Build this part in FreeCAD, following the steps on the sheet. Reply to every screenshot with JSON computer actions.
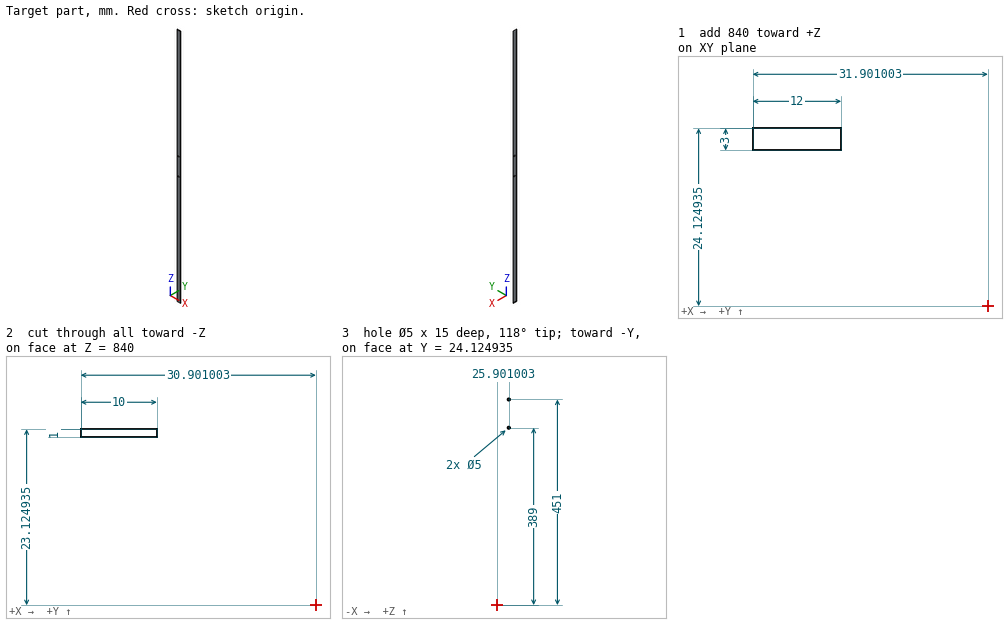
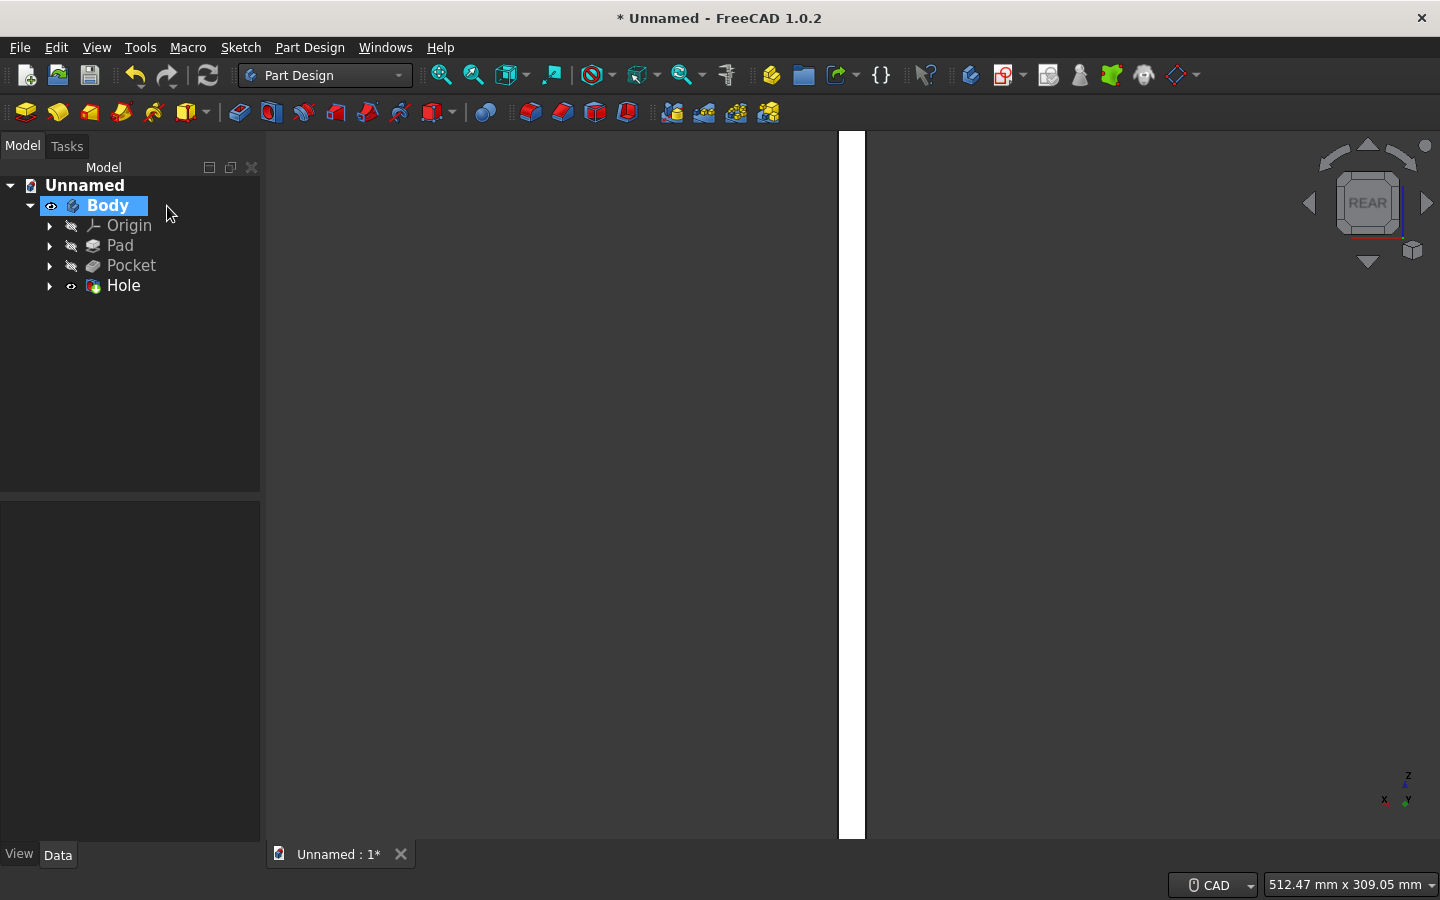
{"action": "key", "text": "0"}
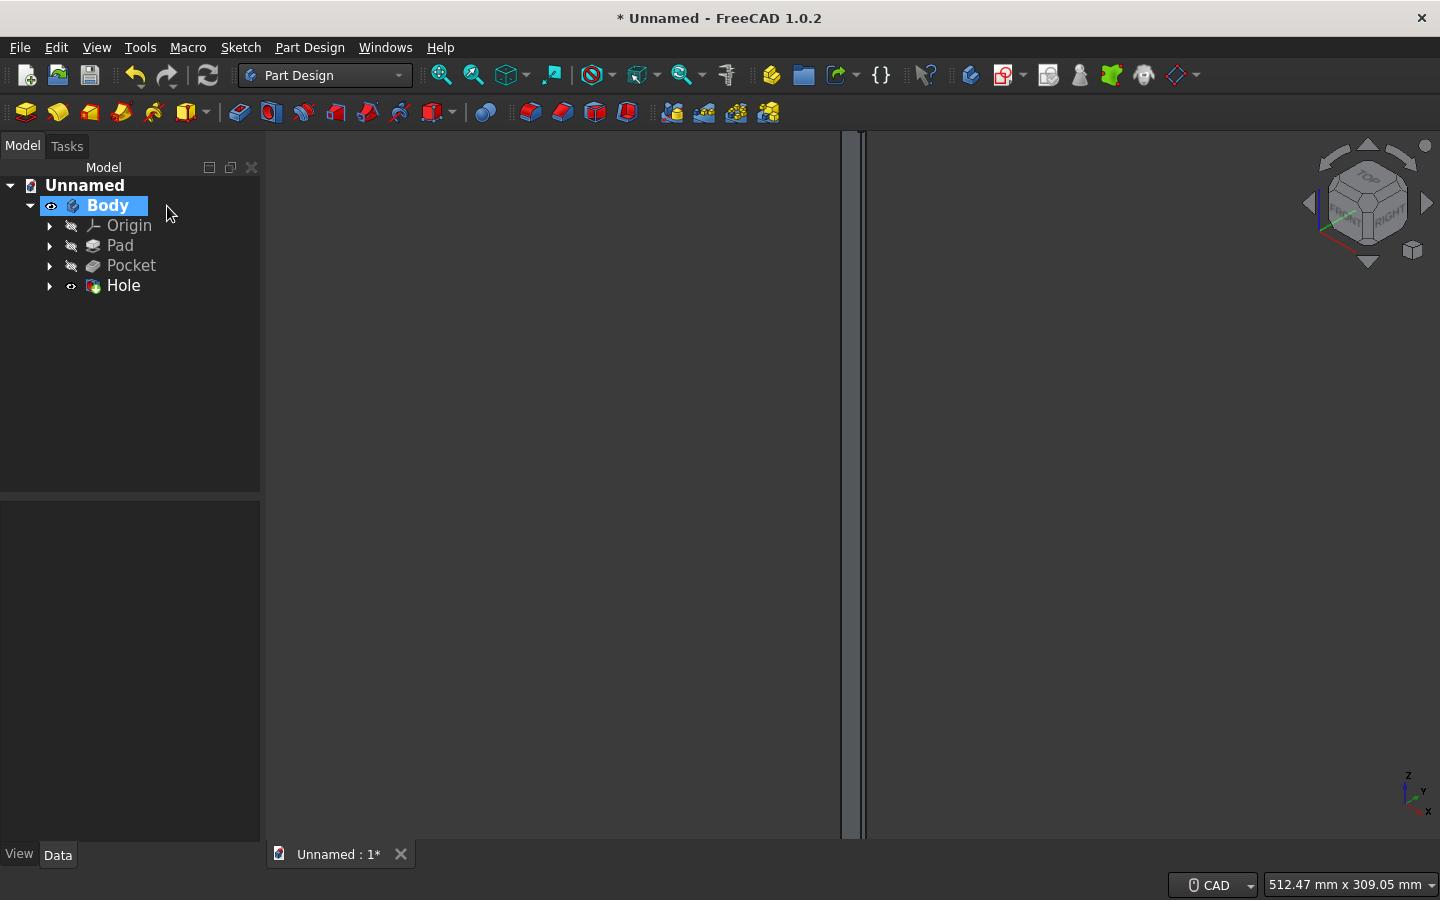
{"action": "key", "text": "v f"}